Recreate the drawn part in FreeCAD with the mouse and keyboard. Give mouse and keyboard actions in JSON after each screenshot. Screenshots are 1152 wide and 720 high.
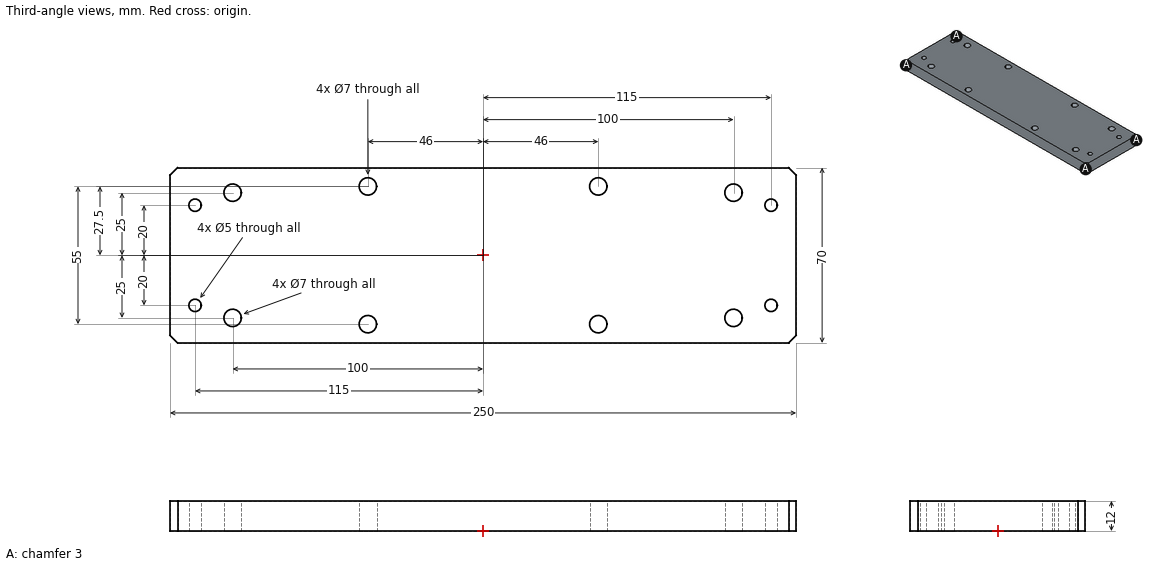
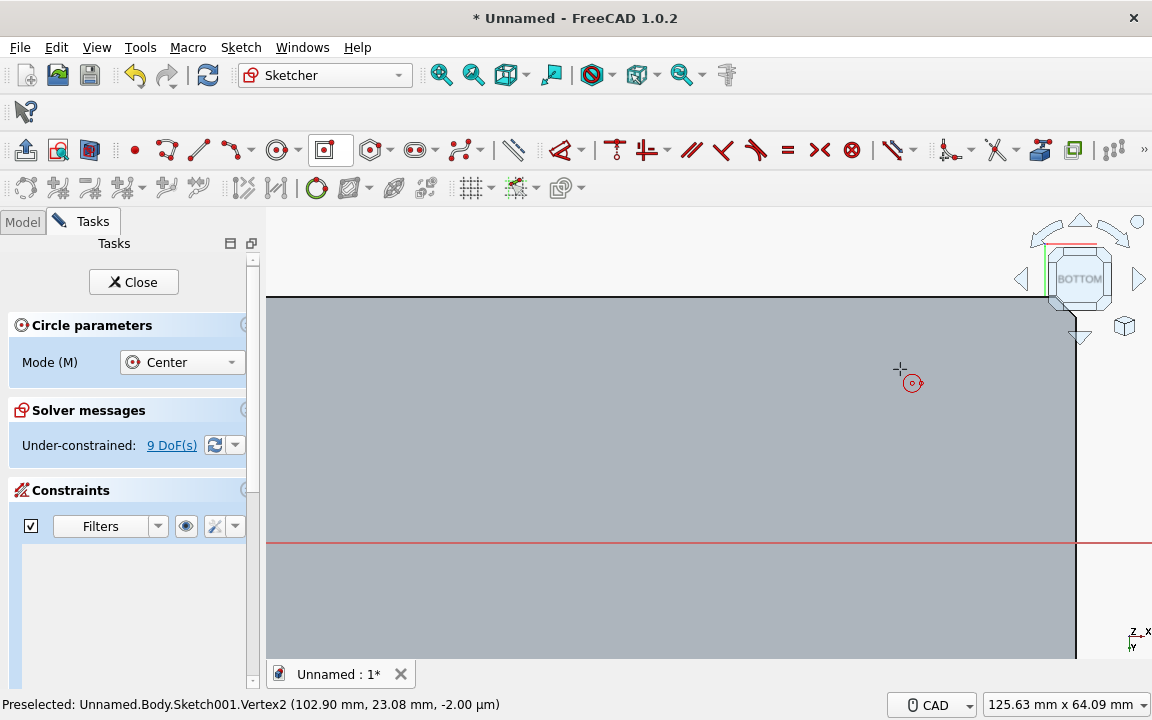
{"action": "left_click", "coordinate": [900, 367]}
{"action": "left_click", "coordinate": [917, 350]}
{"action": "key", "text": "Escape"}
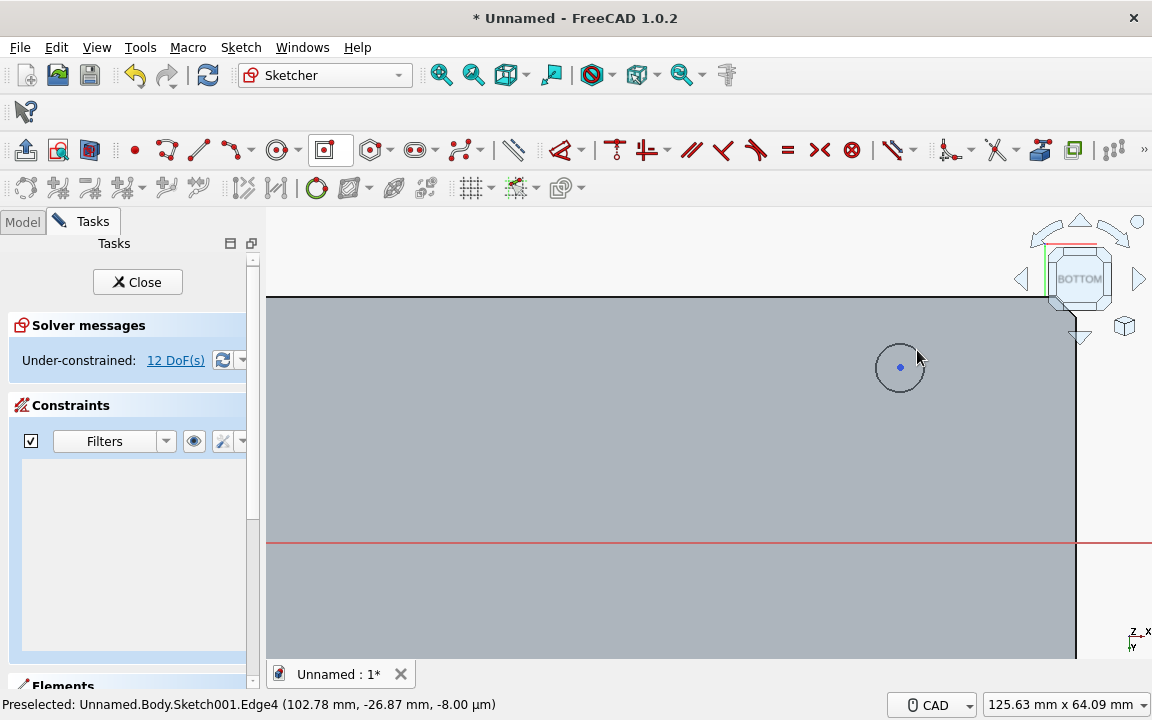
{"action": "scroll", "coordinate": [900, 369], "scroll_direction": "down", "scroll_amount": 5}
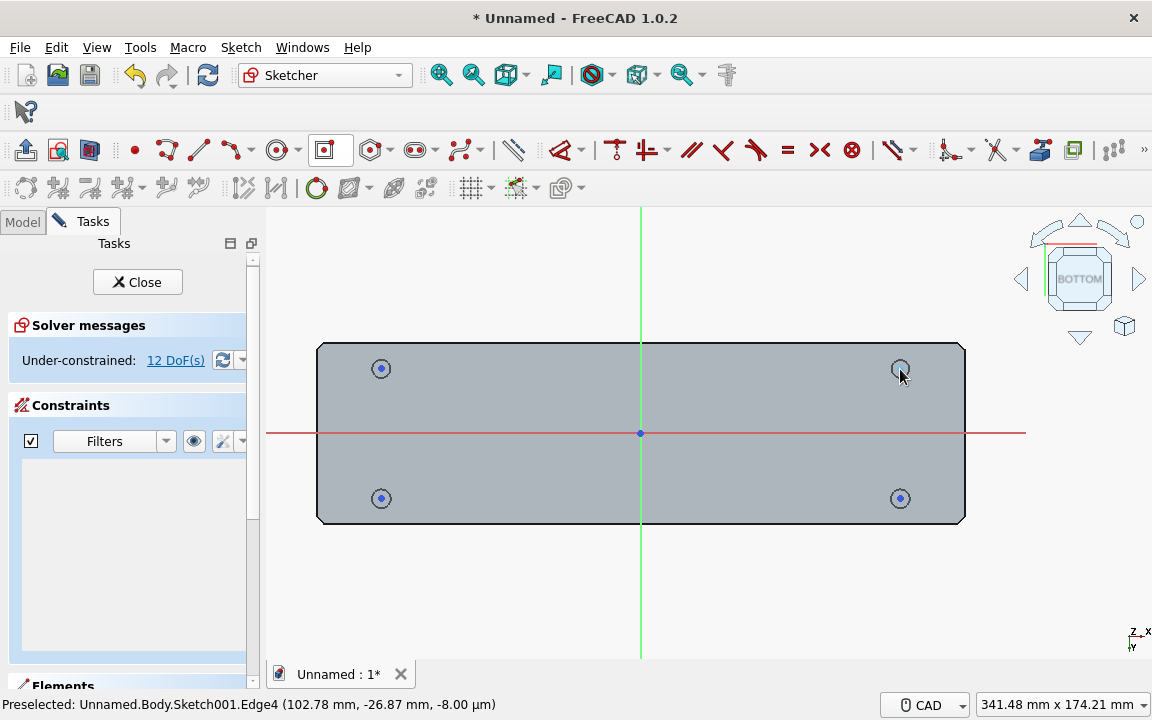
{"action": "scroll", "coordinate": [388, 362], "scroll_direction": "up", "scroll_amount": 3}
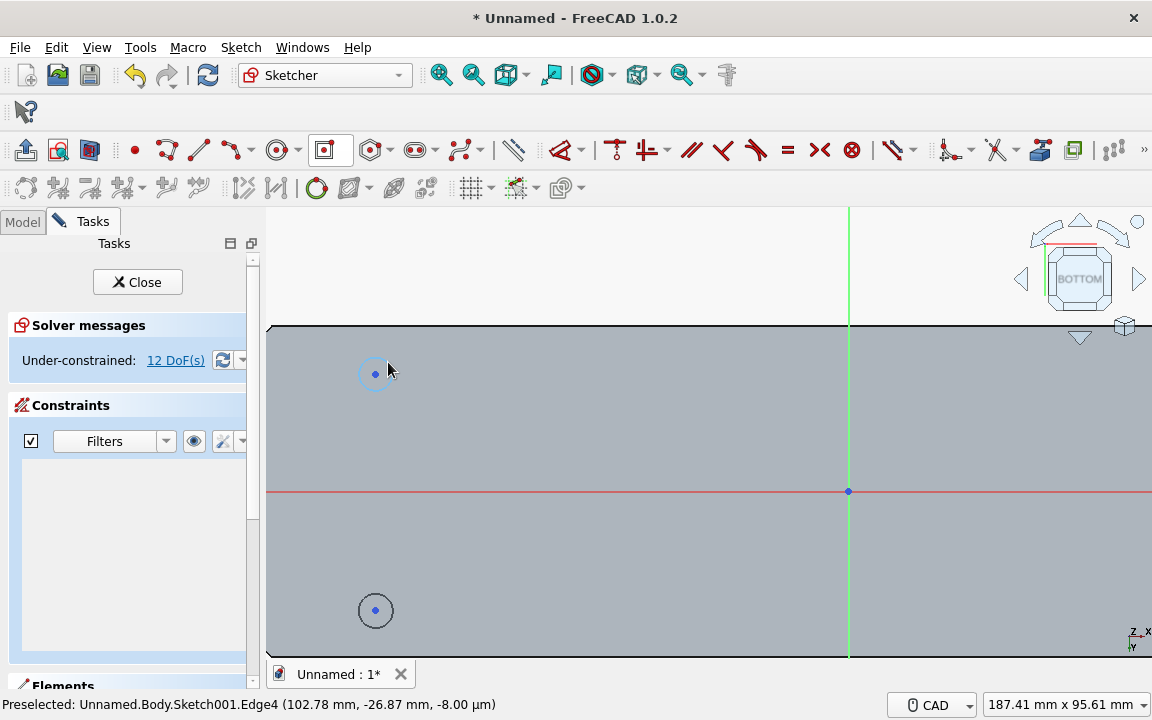
{"action": "left_click", "coordinate": [387, 362]}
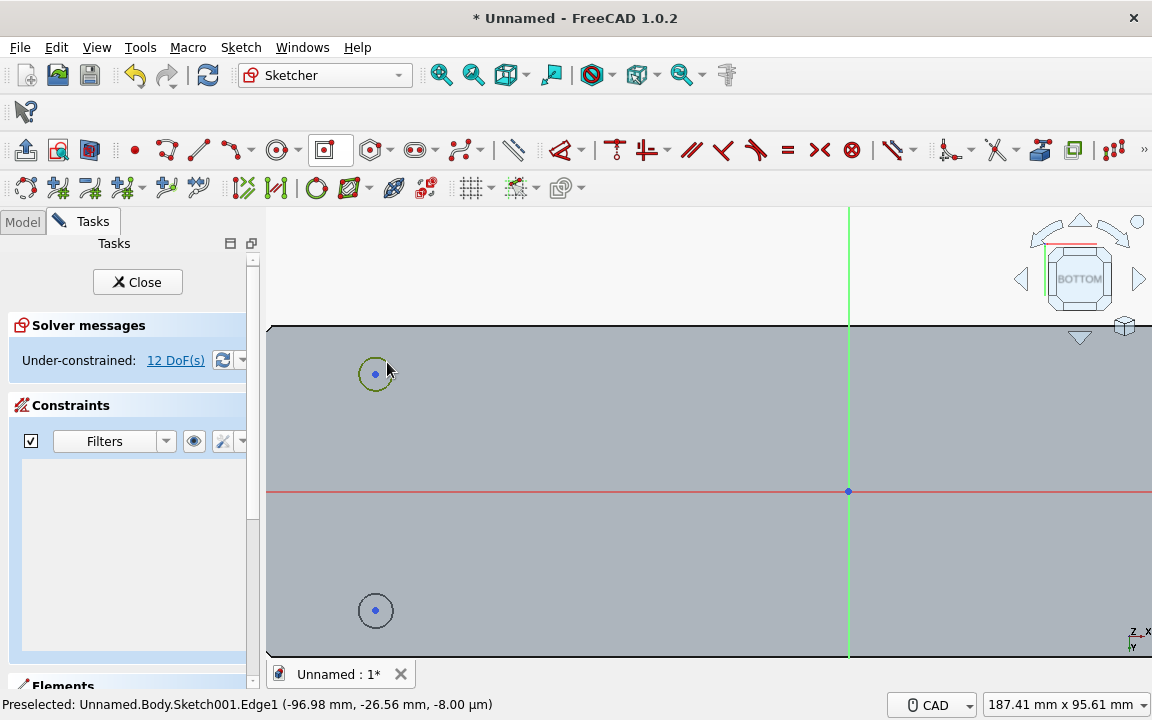
{"action": "left_click", "coordinate": [388, 599]}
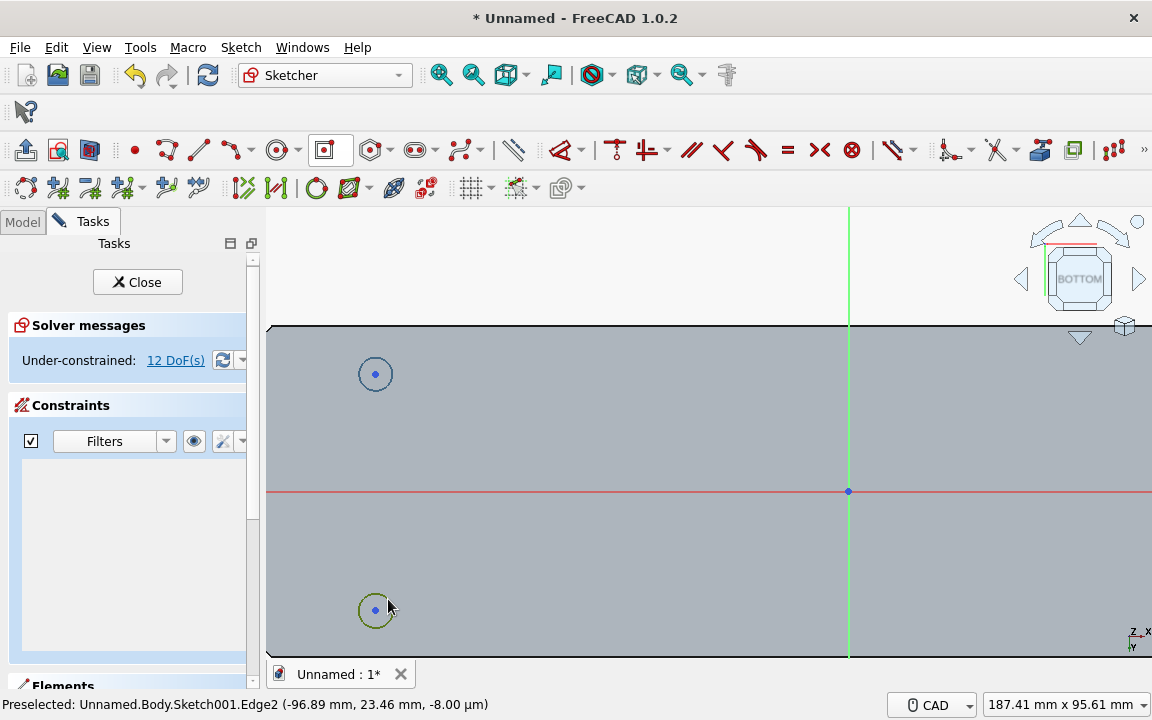
{"action": "scroll", "coordinate": [387, 361], "scroll_direction": "down", "scroll_amount": 3}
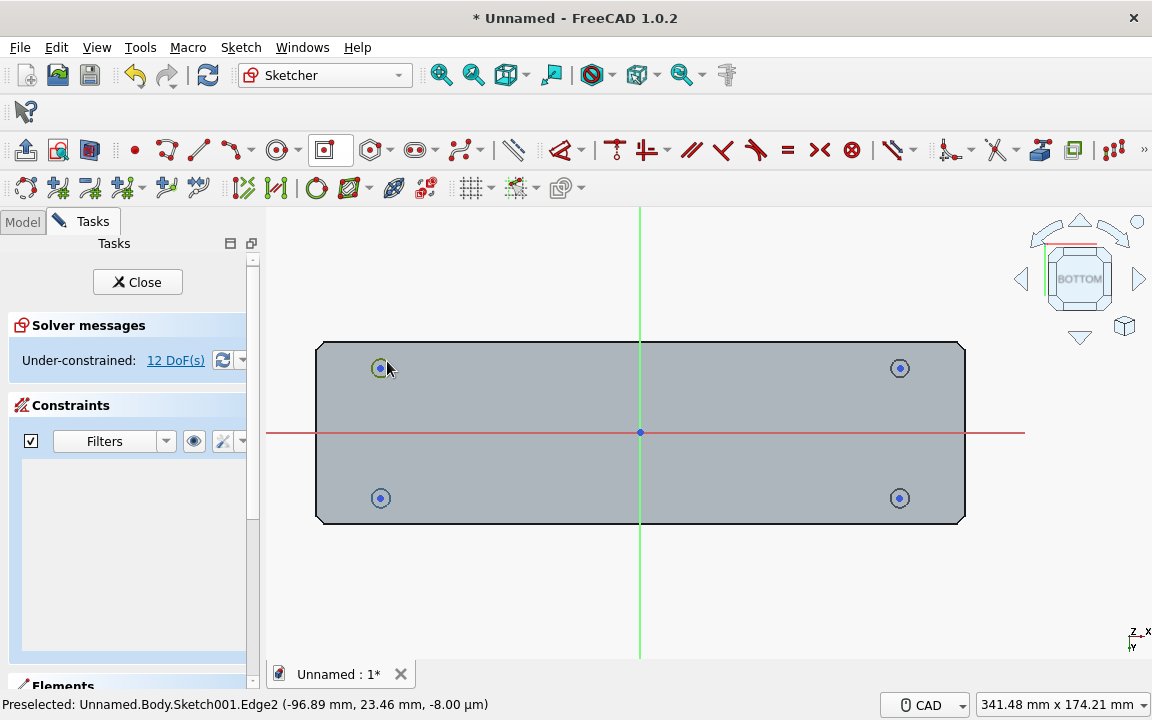
{"action": "scroll", "coordinate": [906, 492], "scroll_direction": "up", "scroll_amount": 2}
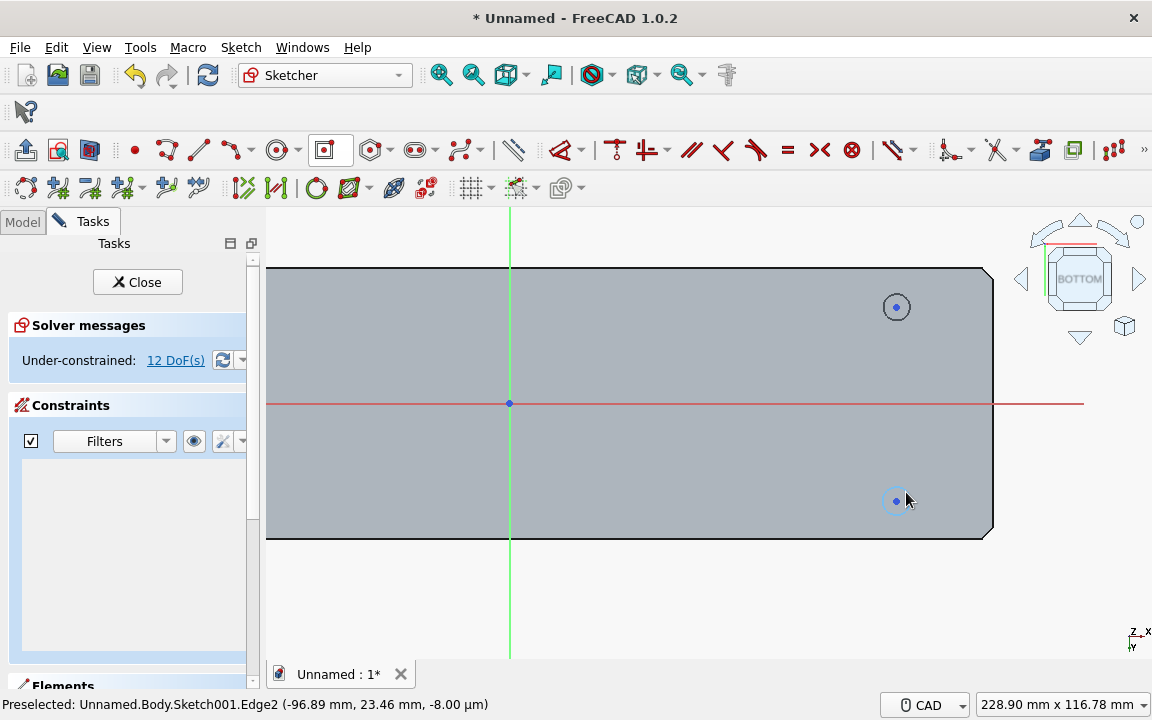
{"action": "left_click", "coordinate": [906, 491]}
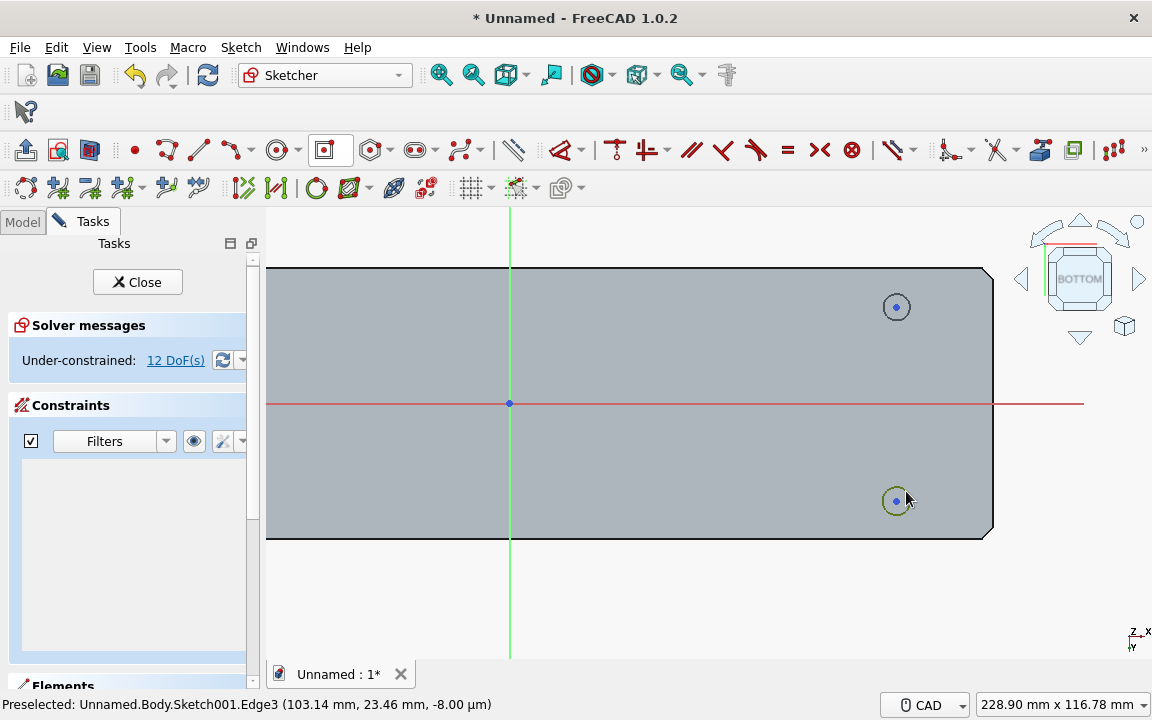
{"action": "left_click", "coordinate": [906, 298]}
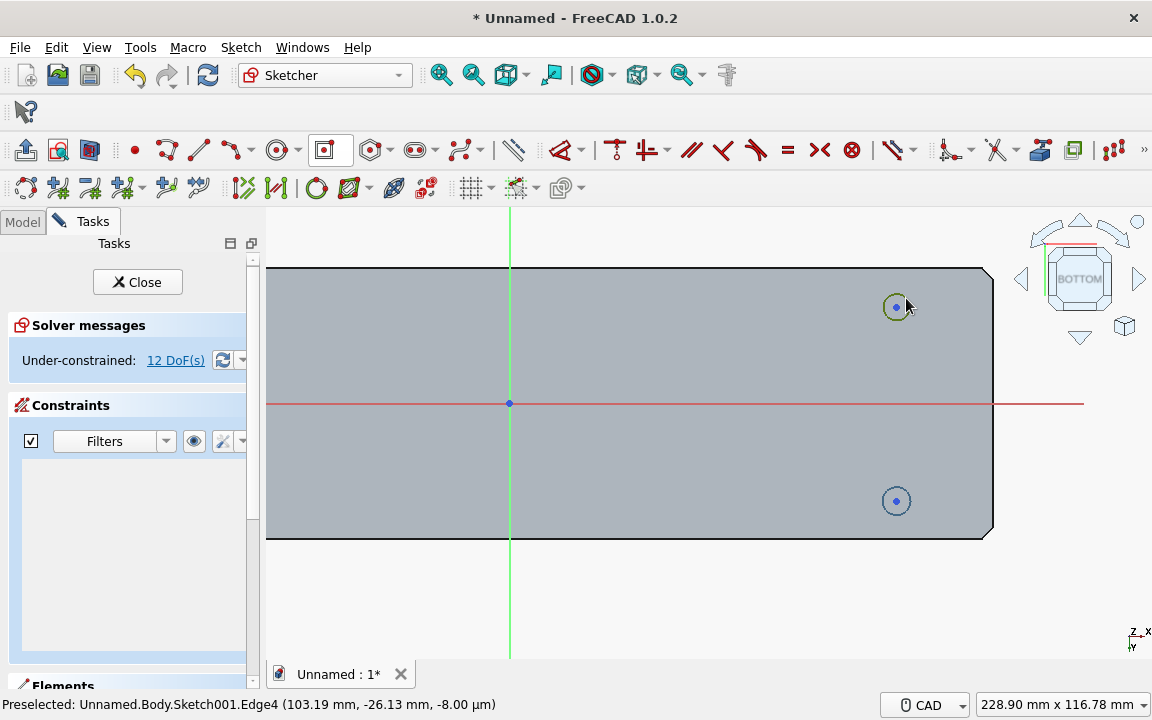
{"action": "left_click", "coordinate": [788, 150]}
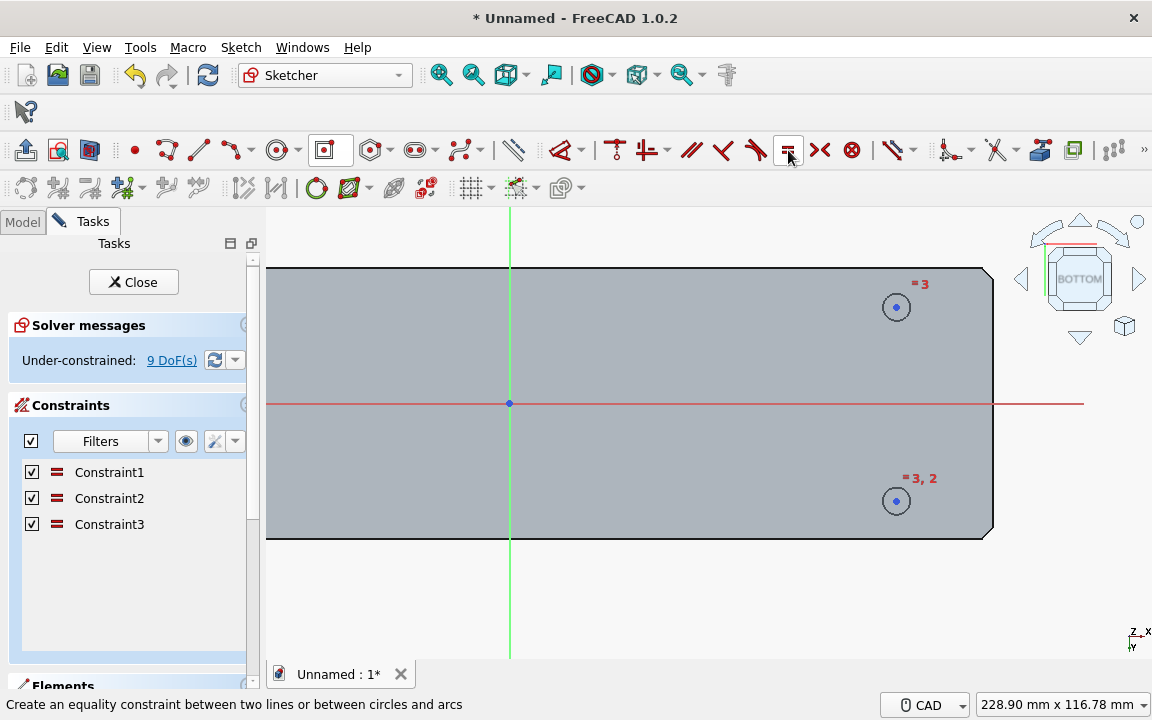
{"action": "scroll", "coordinate": [907, 493], "scroll_direction": "down", "scroll_amount": 2}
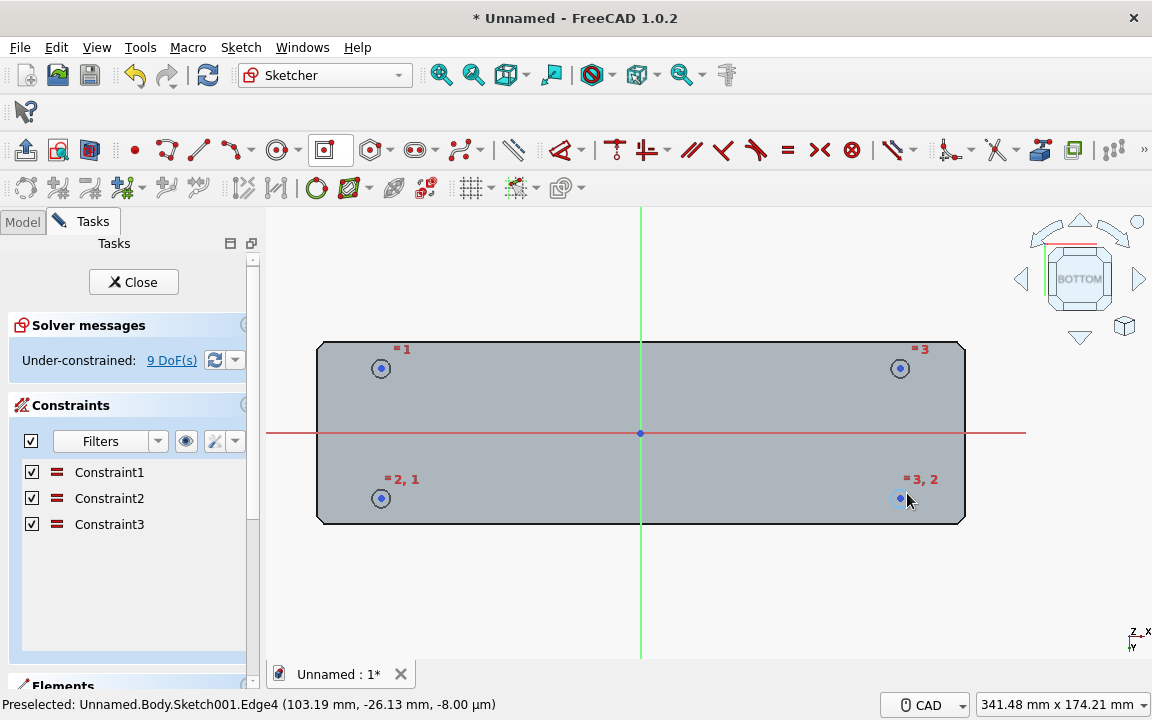
{"action": "left_click", "coordinate": [381, 369]}